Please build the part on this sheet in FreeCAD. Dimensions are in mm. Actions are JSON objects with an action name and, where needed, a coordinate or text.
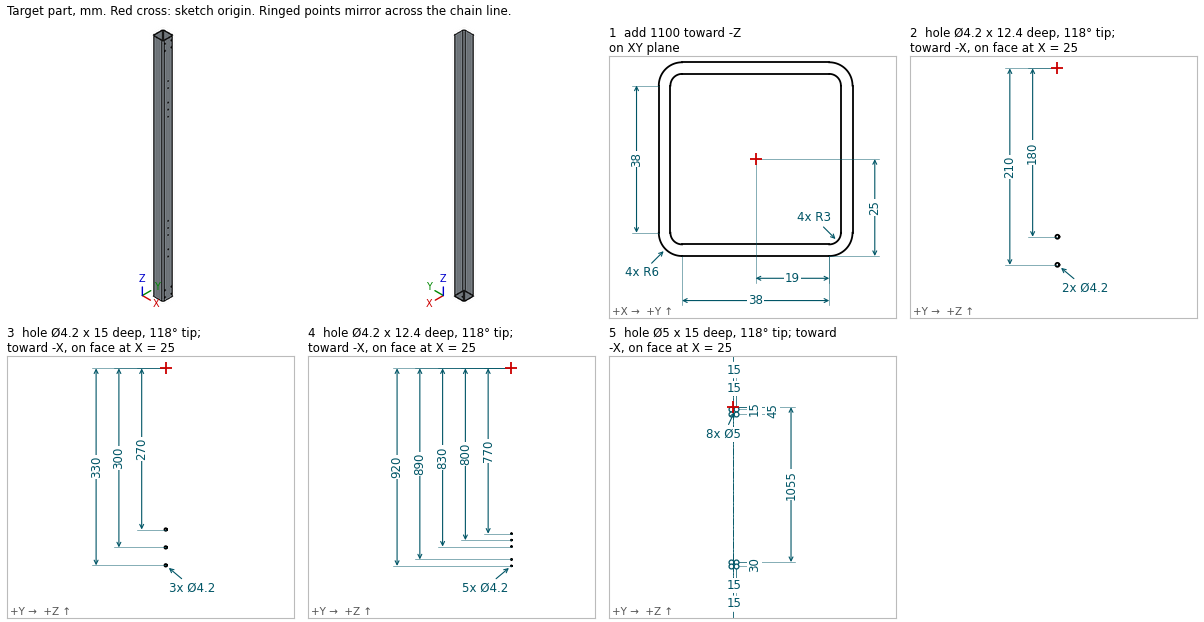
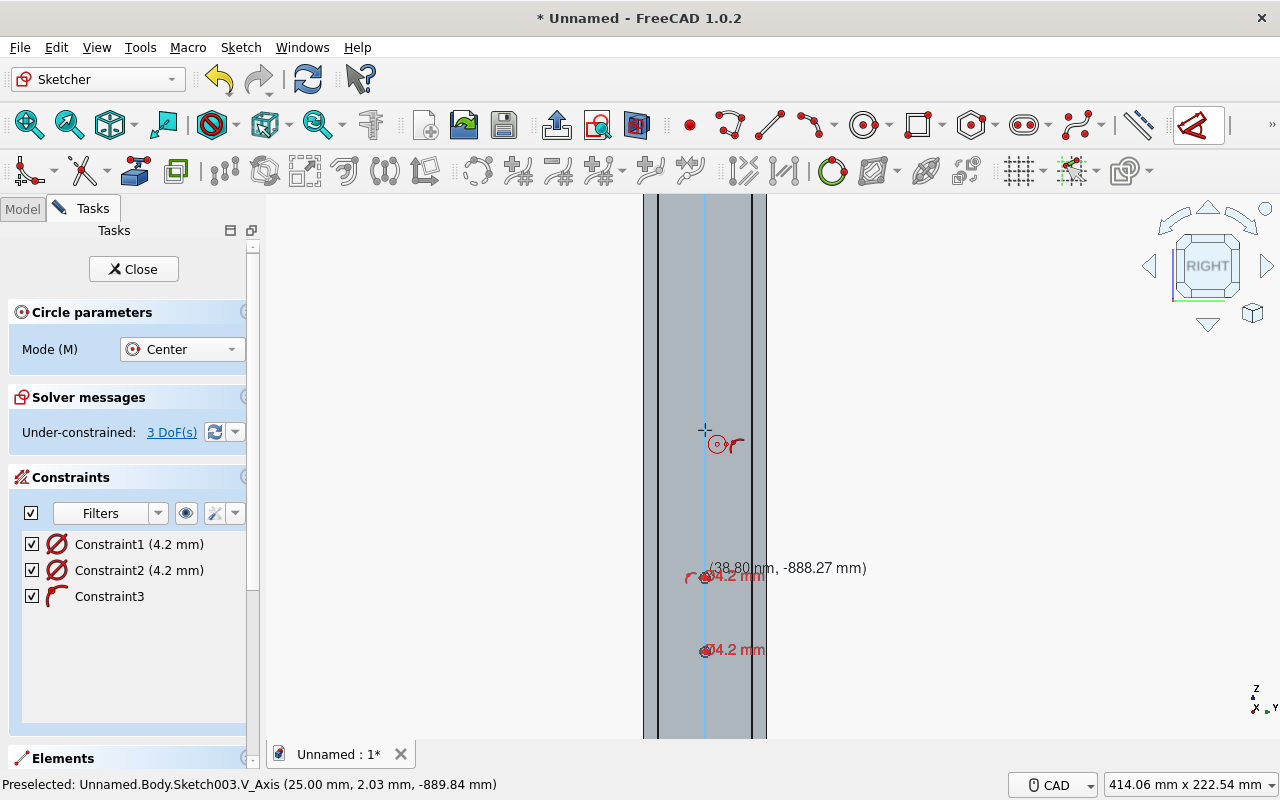
{"action": "left_click", "coordinate": [705, 430]}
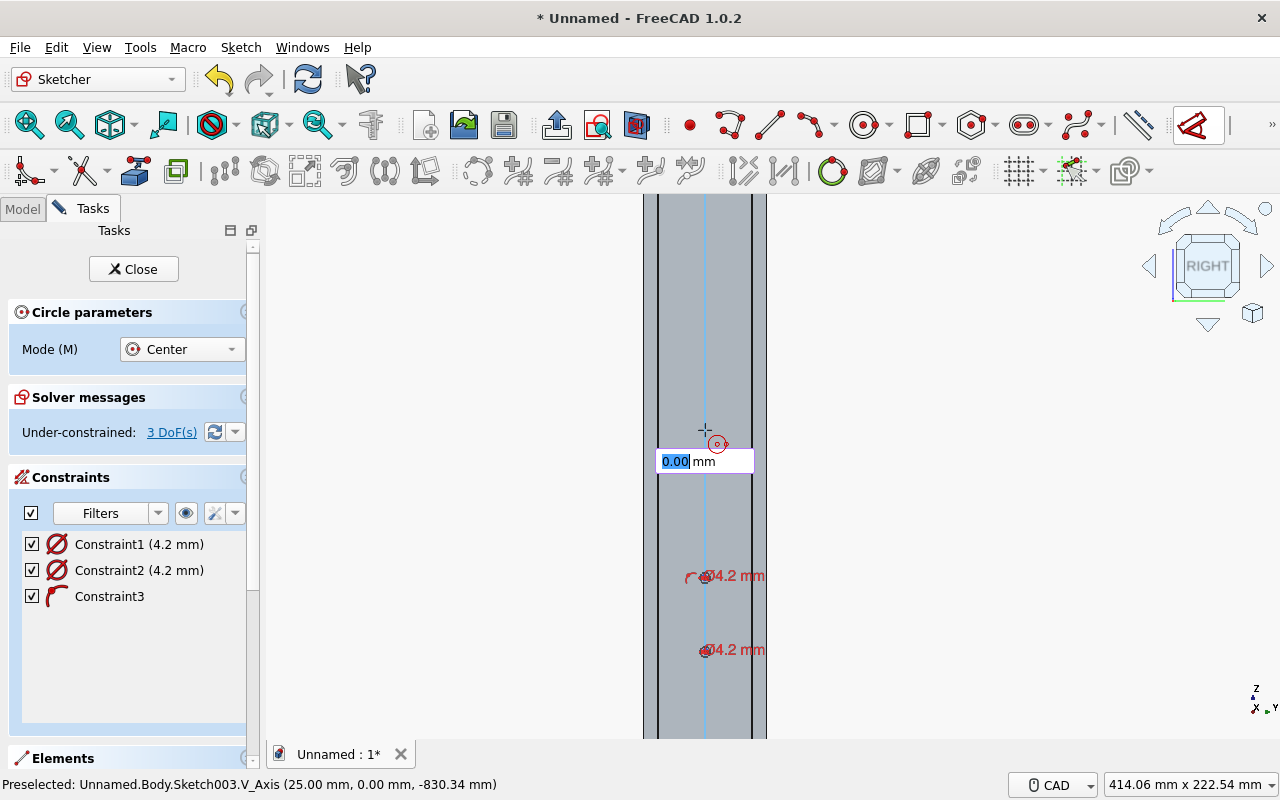
{"action": "scroll", "coordinate": [710, 428], "scroll_direction": "up", "scroll_amount": 6}
{"action": "mouse_move", "coordinate": [708, 428]}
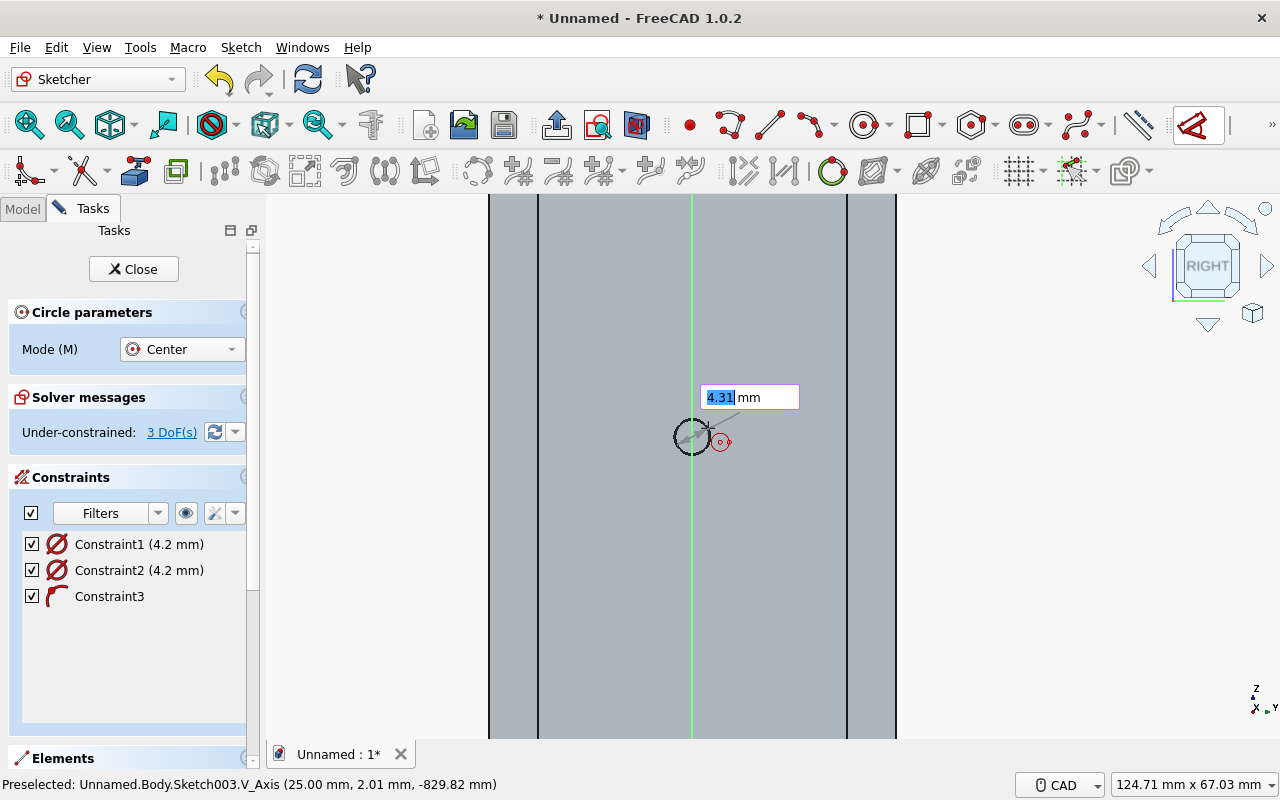
{"action": "type", "text": "4.2"}
{"action": "key", "text": "Return"}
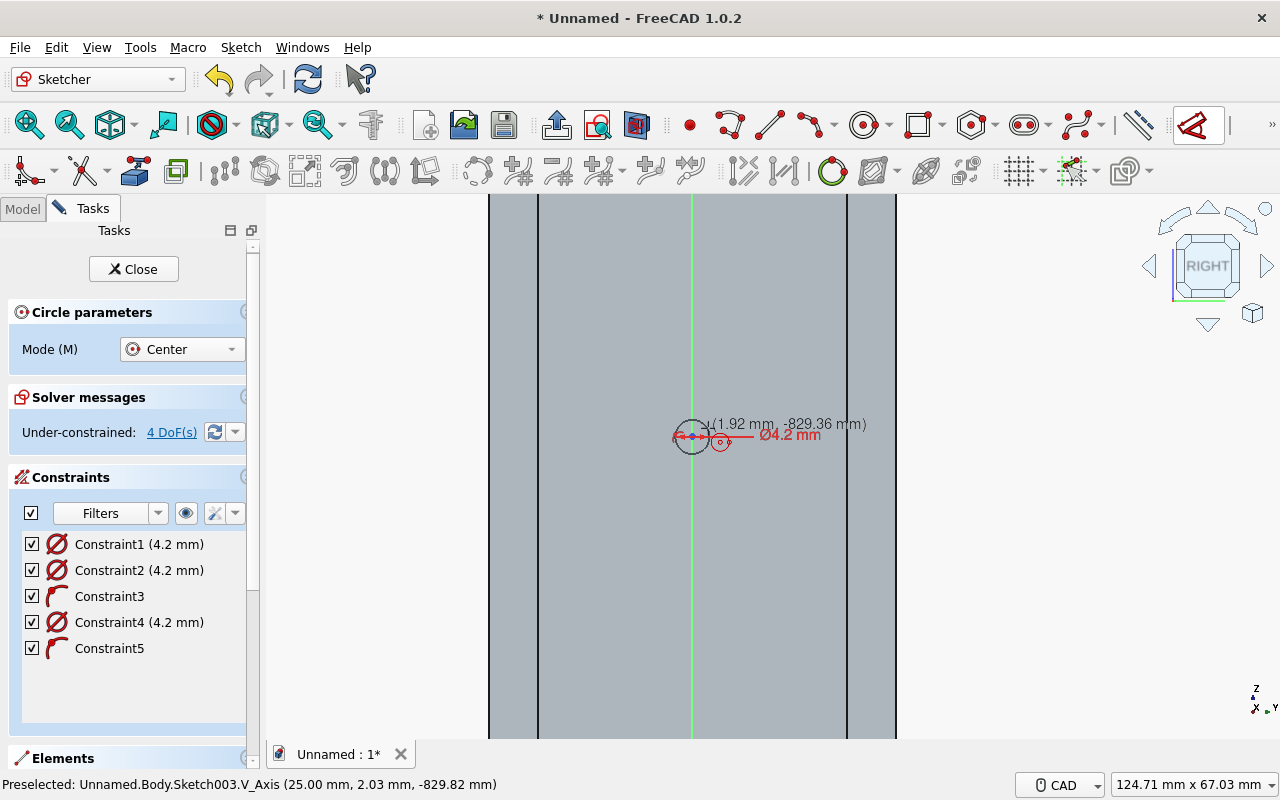
{"action": "scroll", "coordinate": [710, 428], "scroll_direction": "down", "scroll_amount": 6}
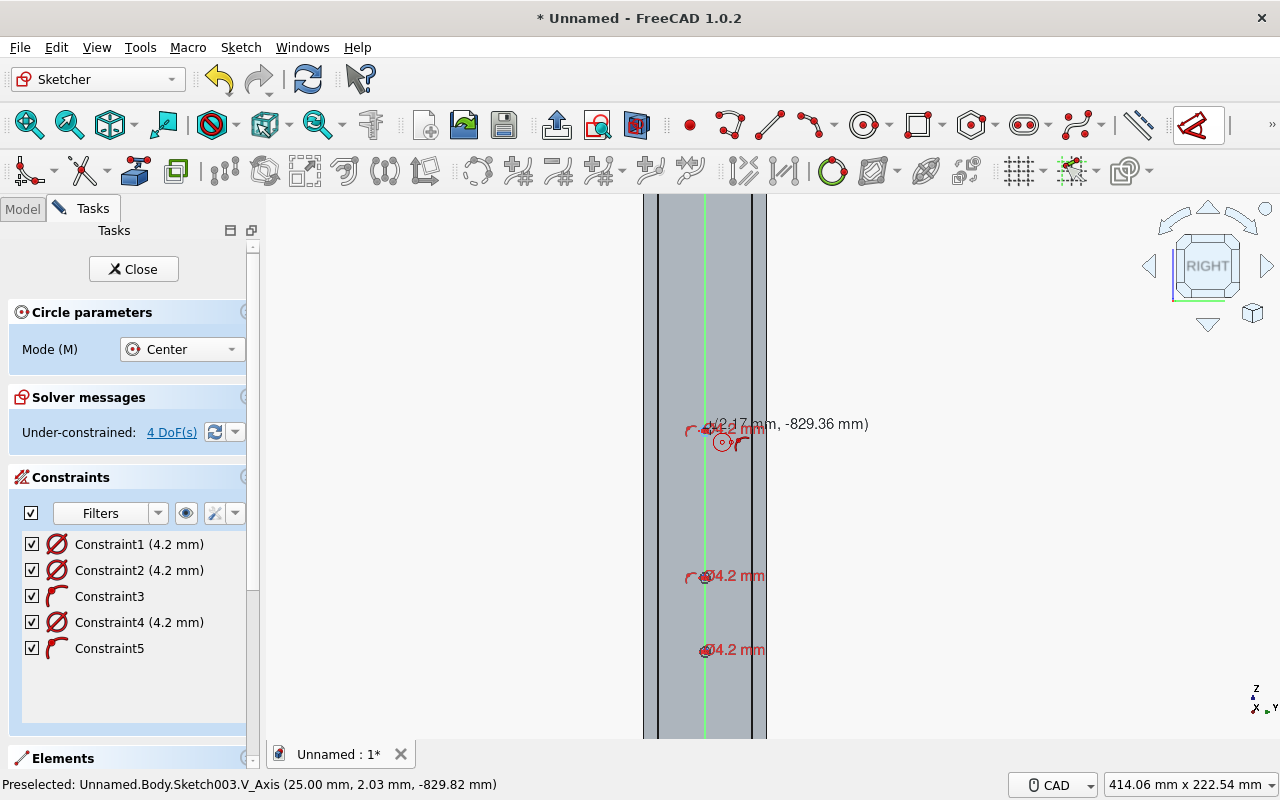
{"action": "scroll", "coordinate": [705, 357], "scroll_direction": "up", "scroll_amount": 8}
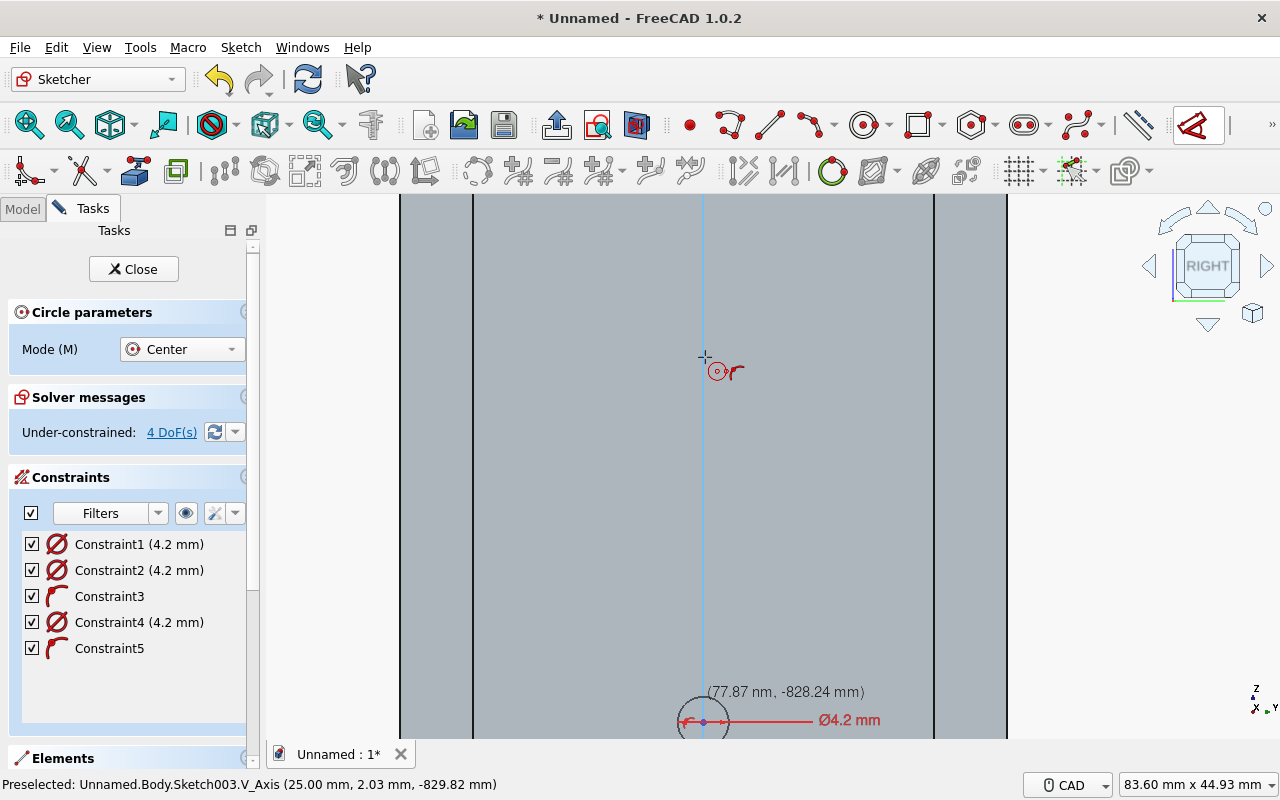
{"action": "scroll", "coordinate": [705, 357], "scroll_direction": "down", "scroll_amount": 8}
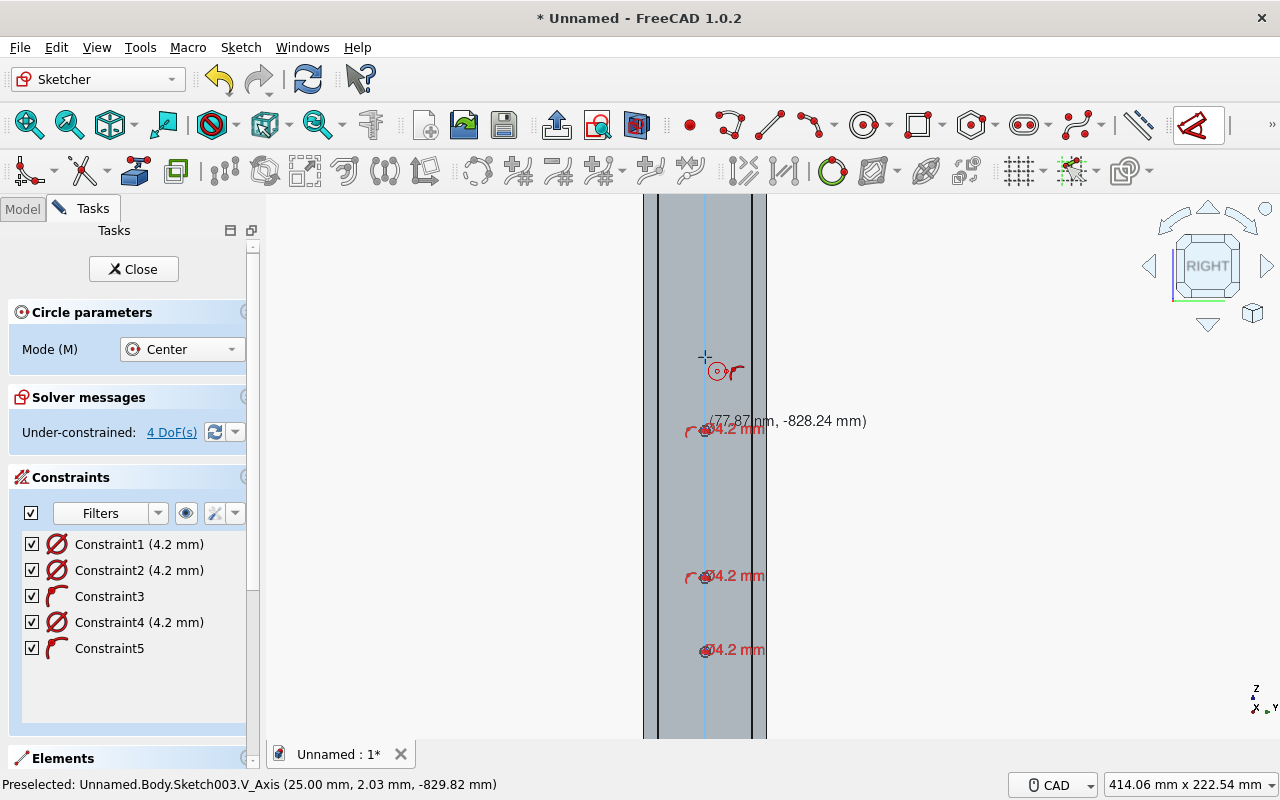
{"action": "left_click", "coordinate": [705, 357]}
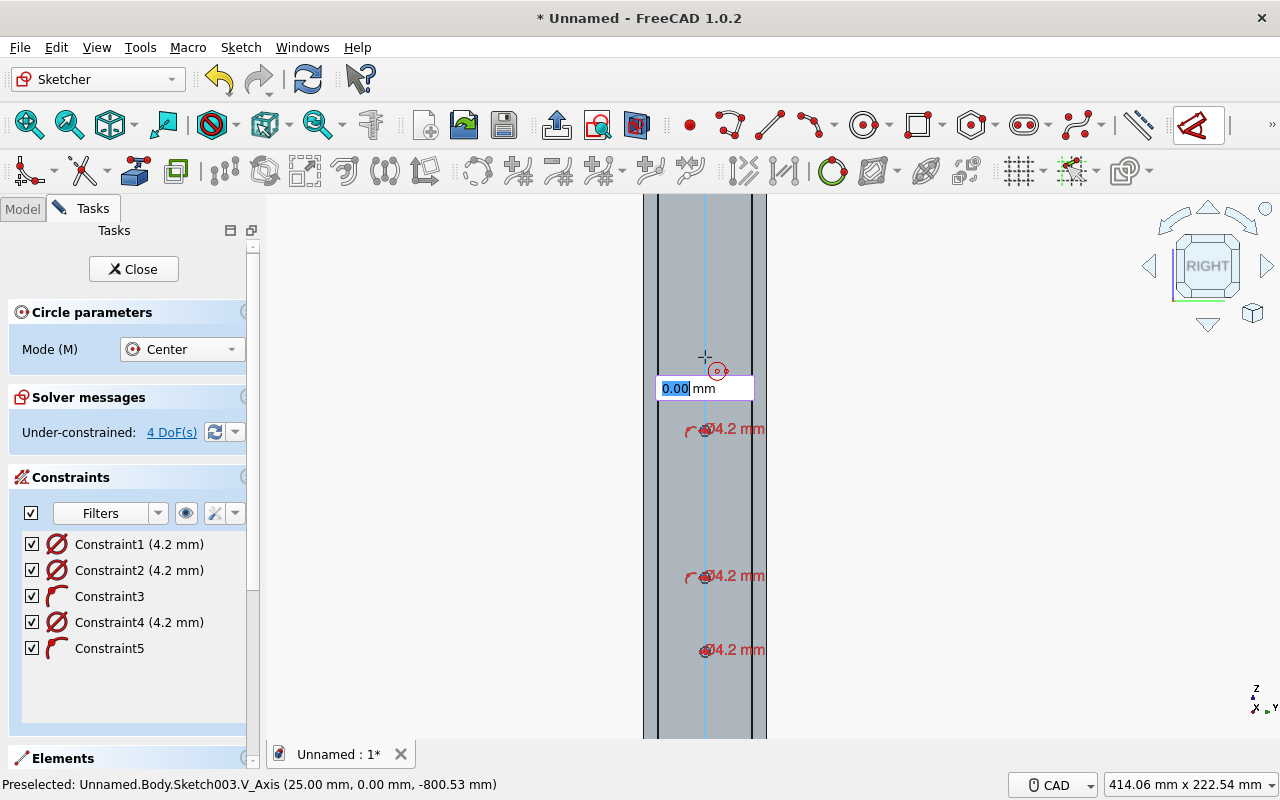
{"action": "scroll", "coordinate": [710, 355], "scroll_direction": "up", "scroll_amount": 6}
{"action": "mouse_move", "coordinate": [708, 354]}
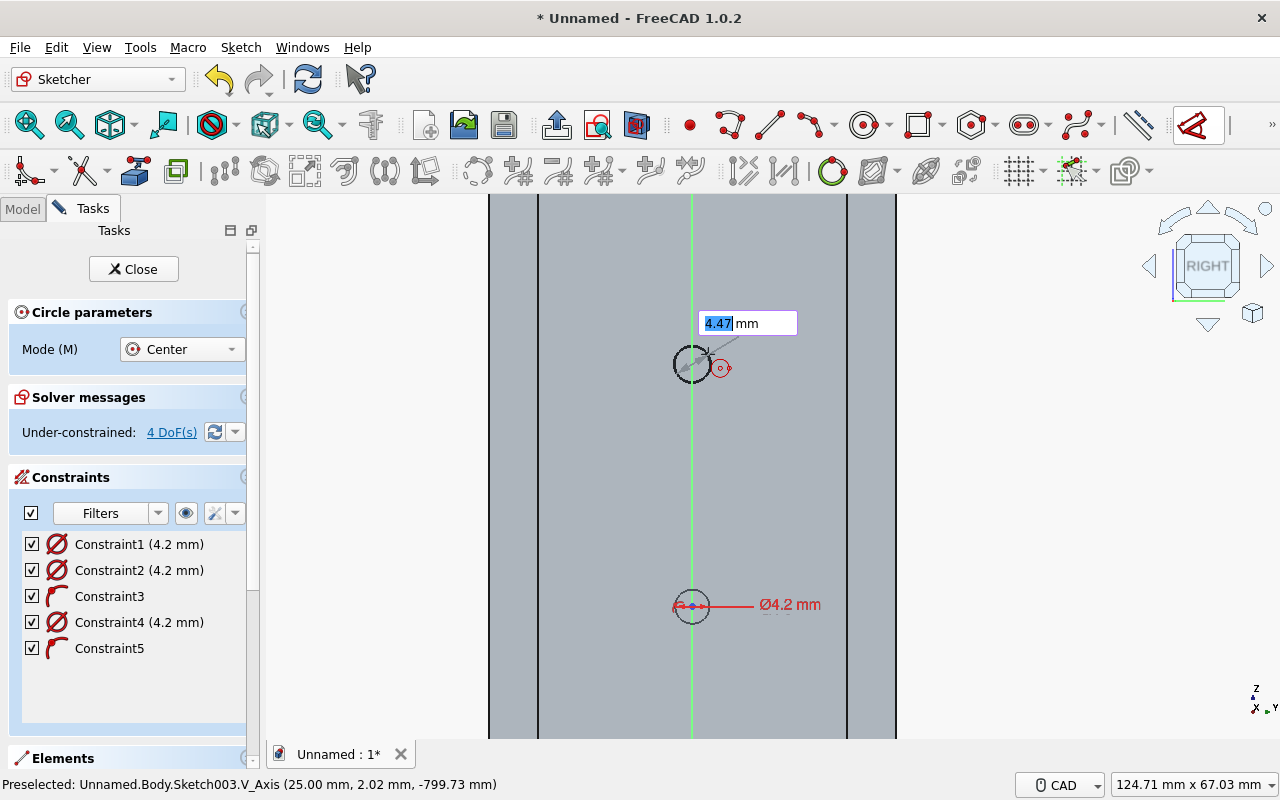
{"action": "type", "text": "4.2"}
{"action": "key", "text": "Return"}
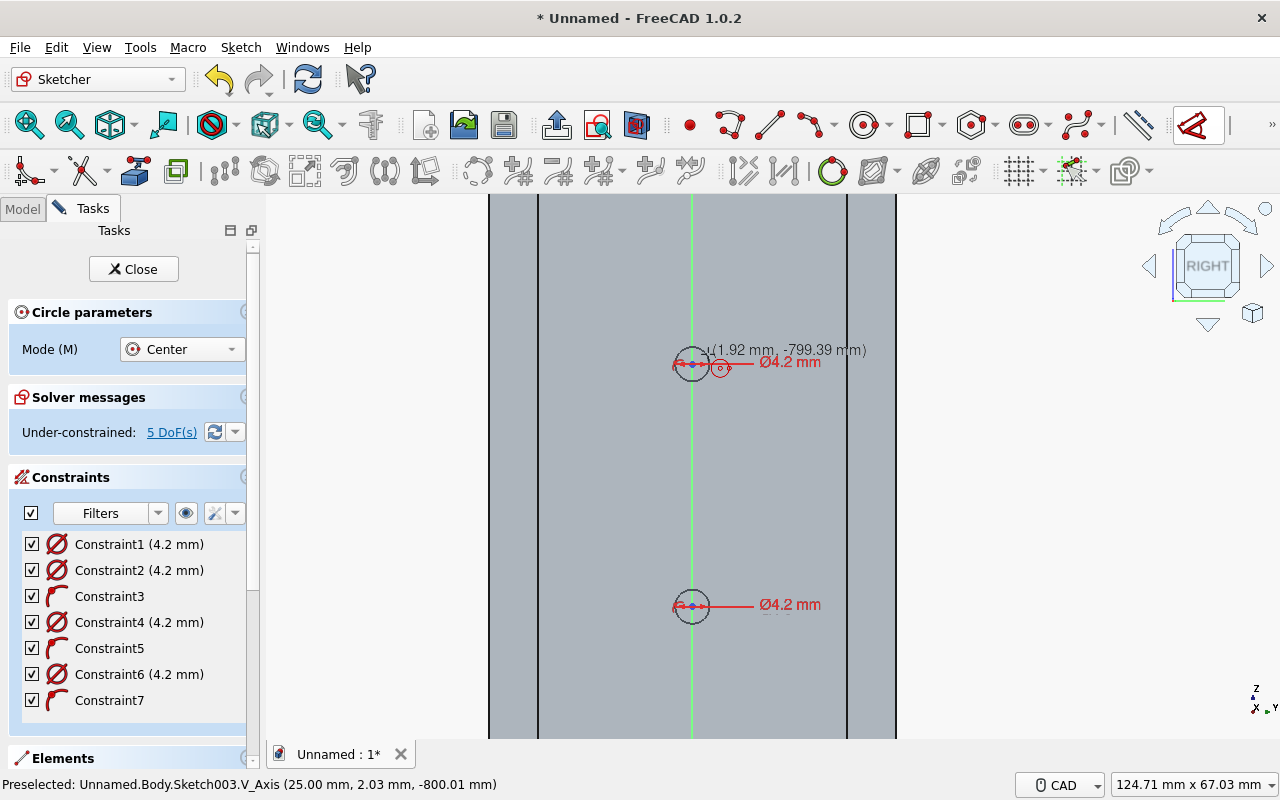
{"action": "scroll", "coordinate": [710, 355], "scroll_direction": "down", "scroll_amount": 6}